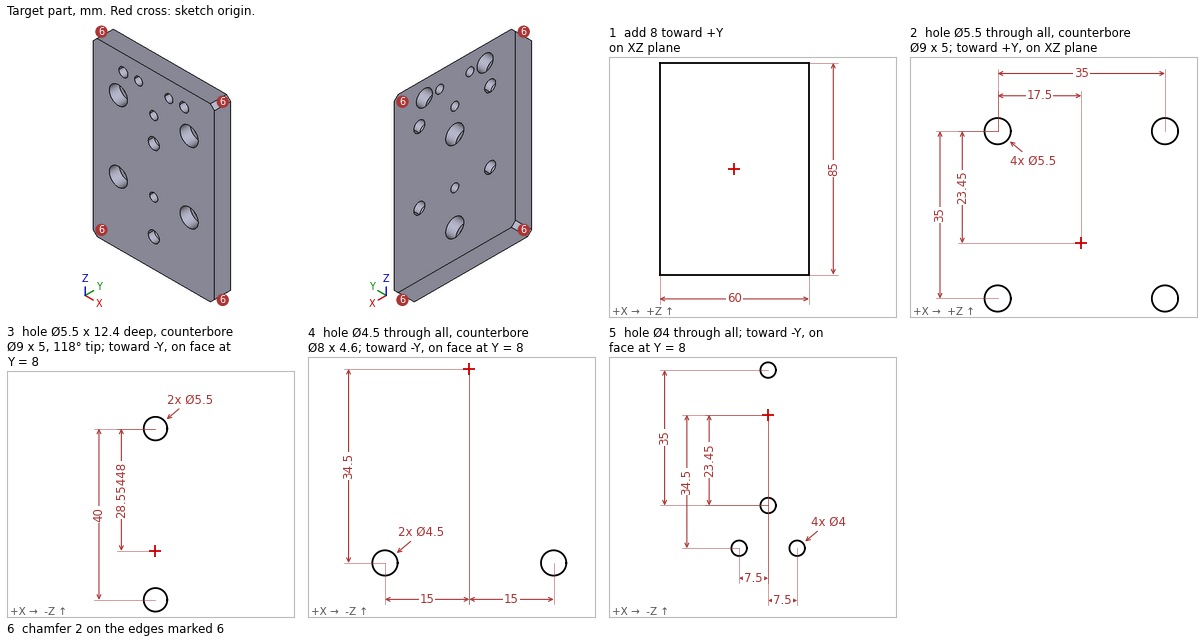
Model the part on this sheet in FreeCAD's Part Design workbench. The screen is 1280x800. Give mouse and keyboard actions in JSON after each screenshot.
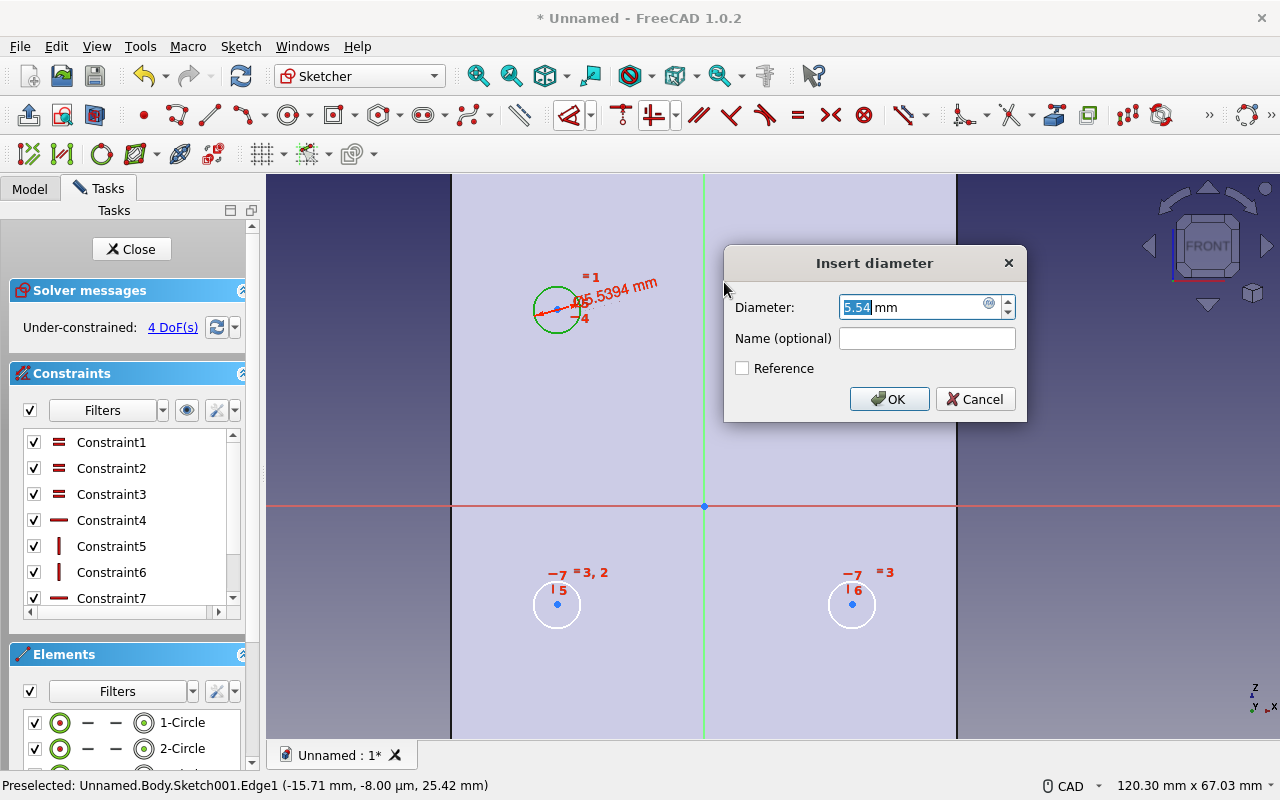
{"action": "type", "text": "5.5"}
{"action": "key", "text": "Return"}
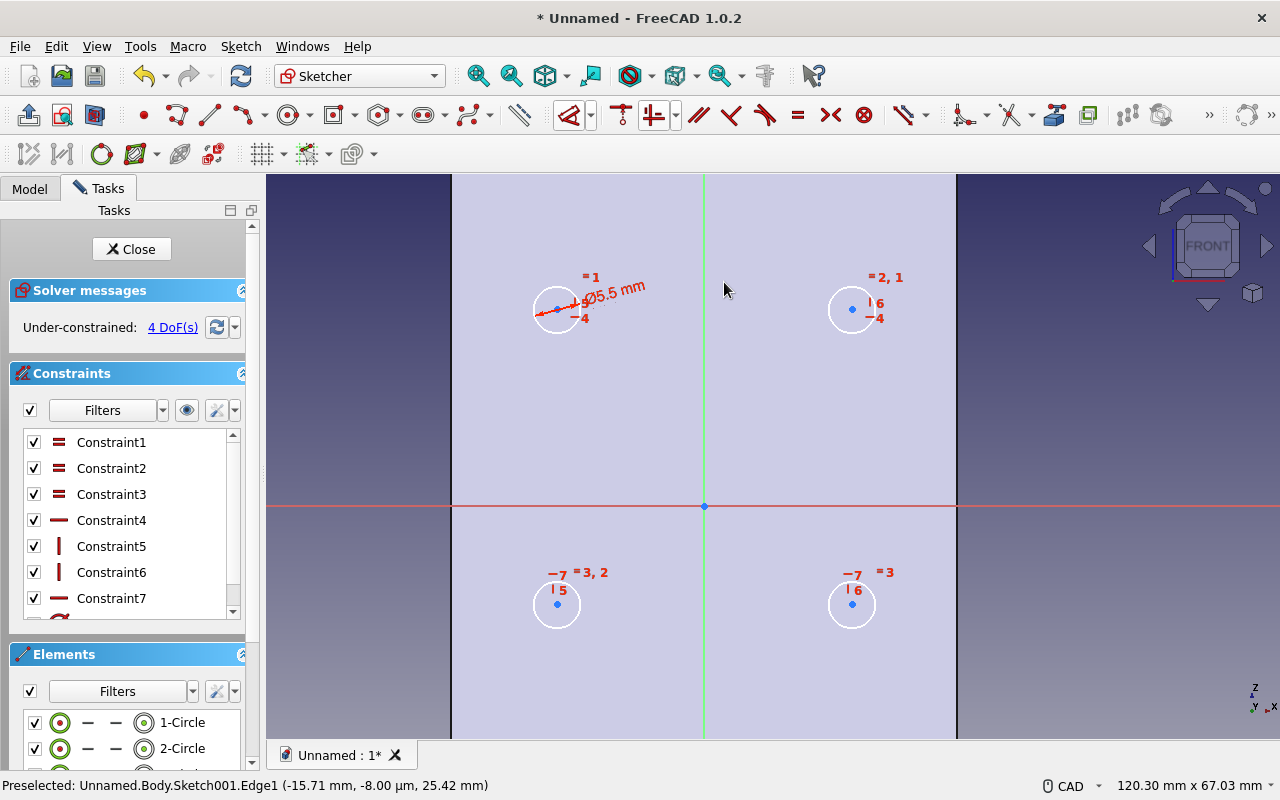
{"action": "left_click", "coordinate": [557, 310]}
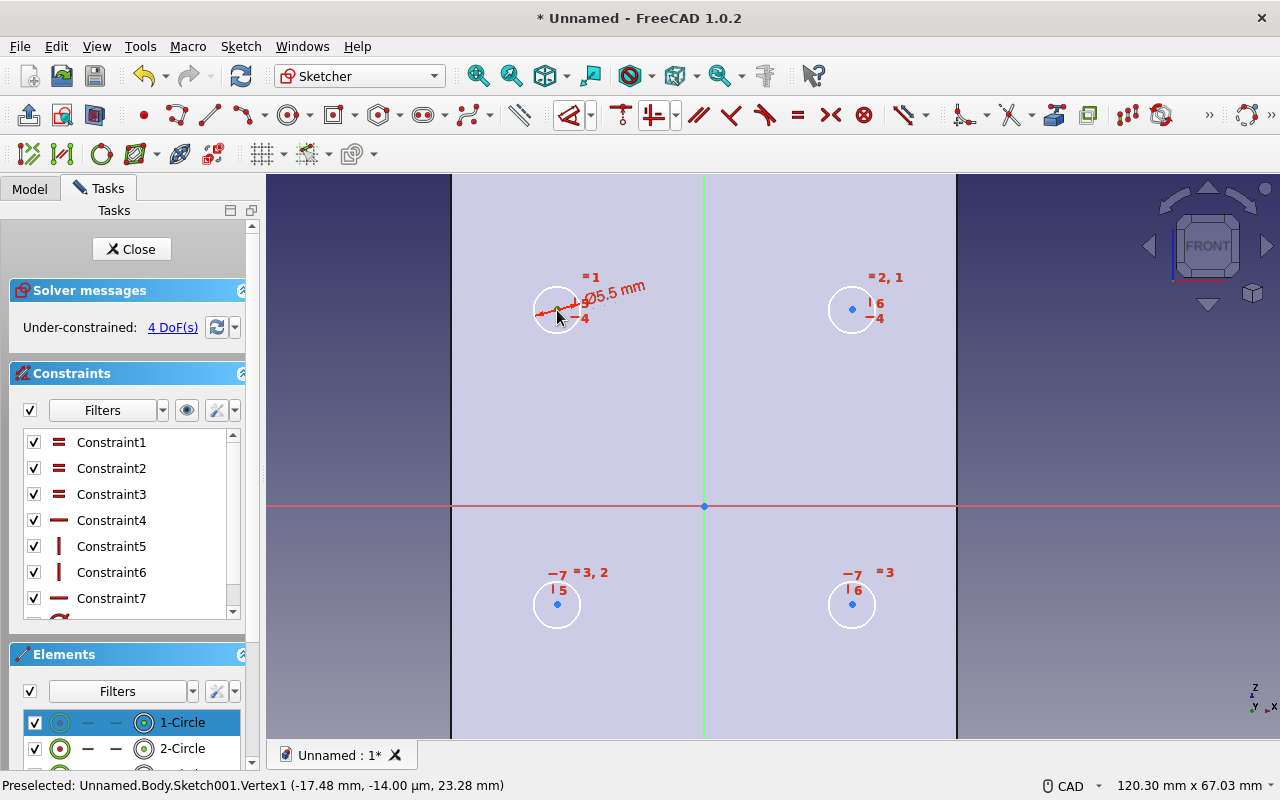
{"action": "left_click", "coordinate": [852, 310]}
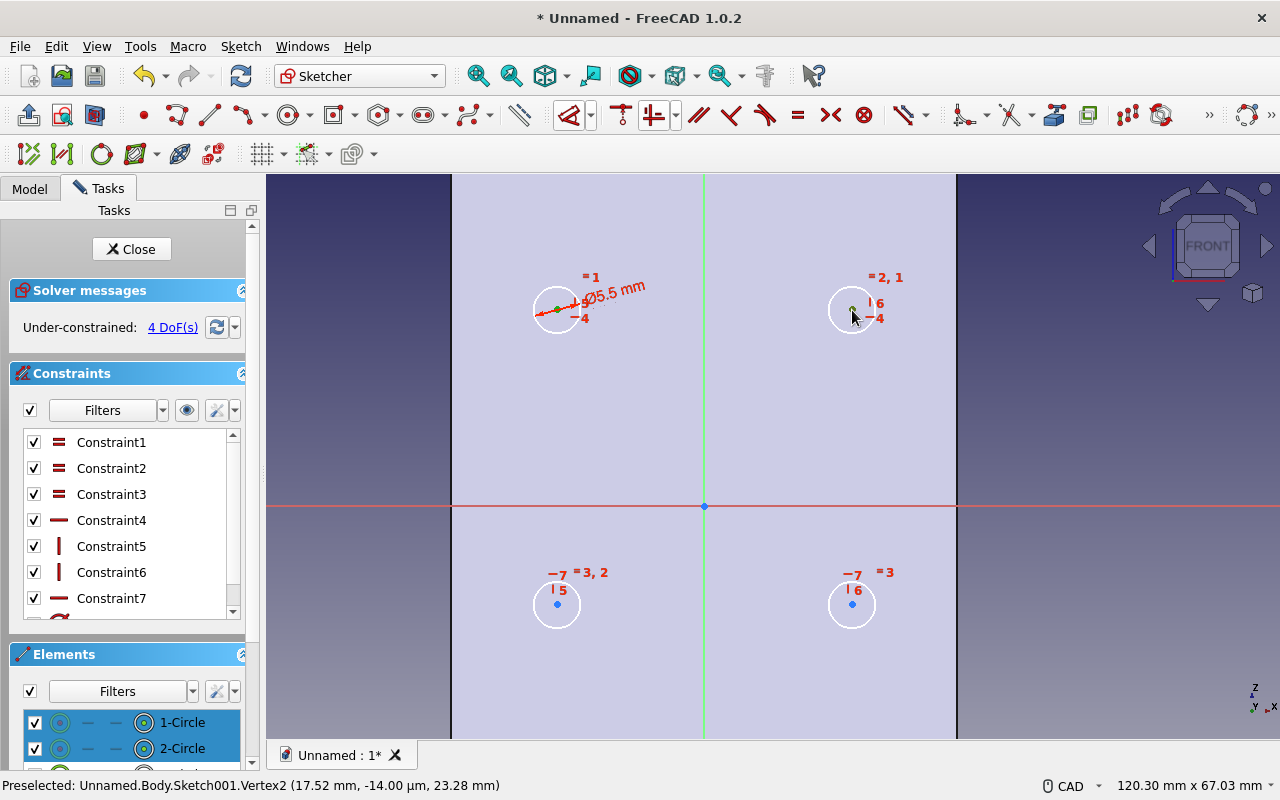
{"action": "key", "text": "l"}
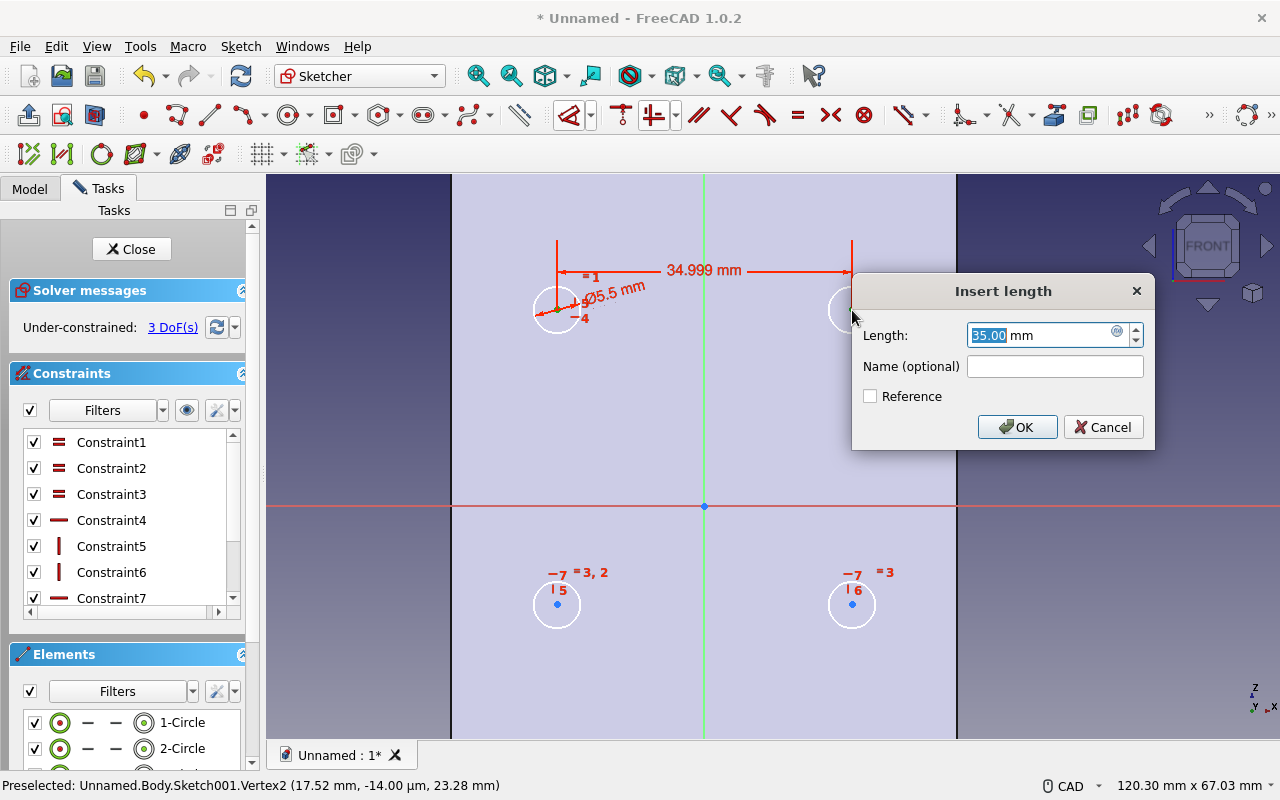
{"action": "type", "text": "35"}
{"action": "key", "text": "Return"}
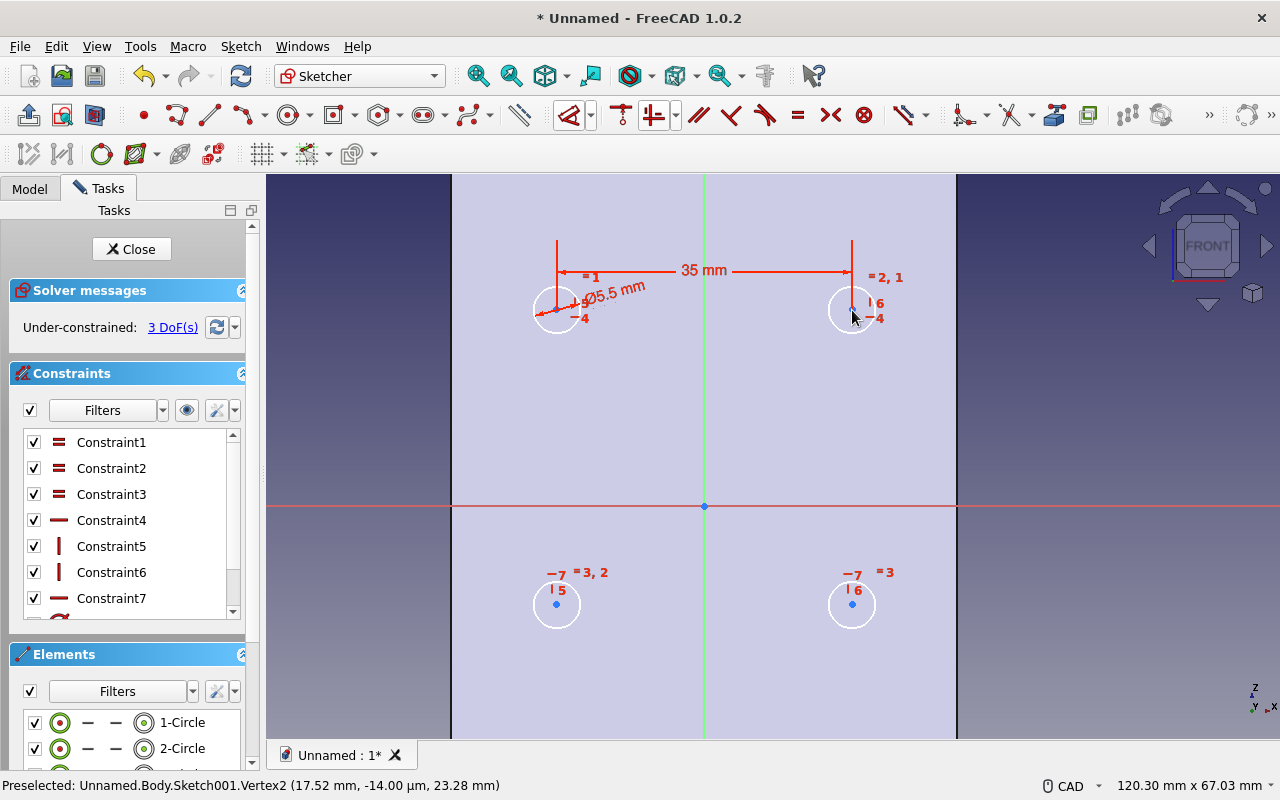
{"action": "left_click", "coordinate": [557, 310]}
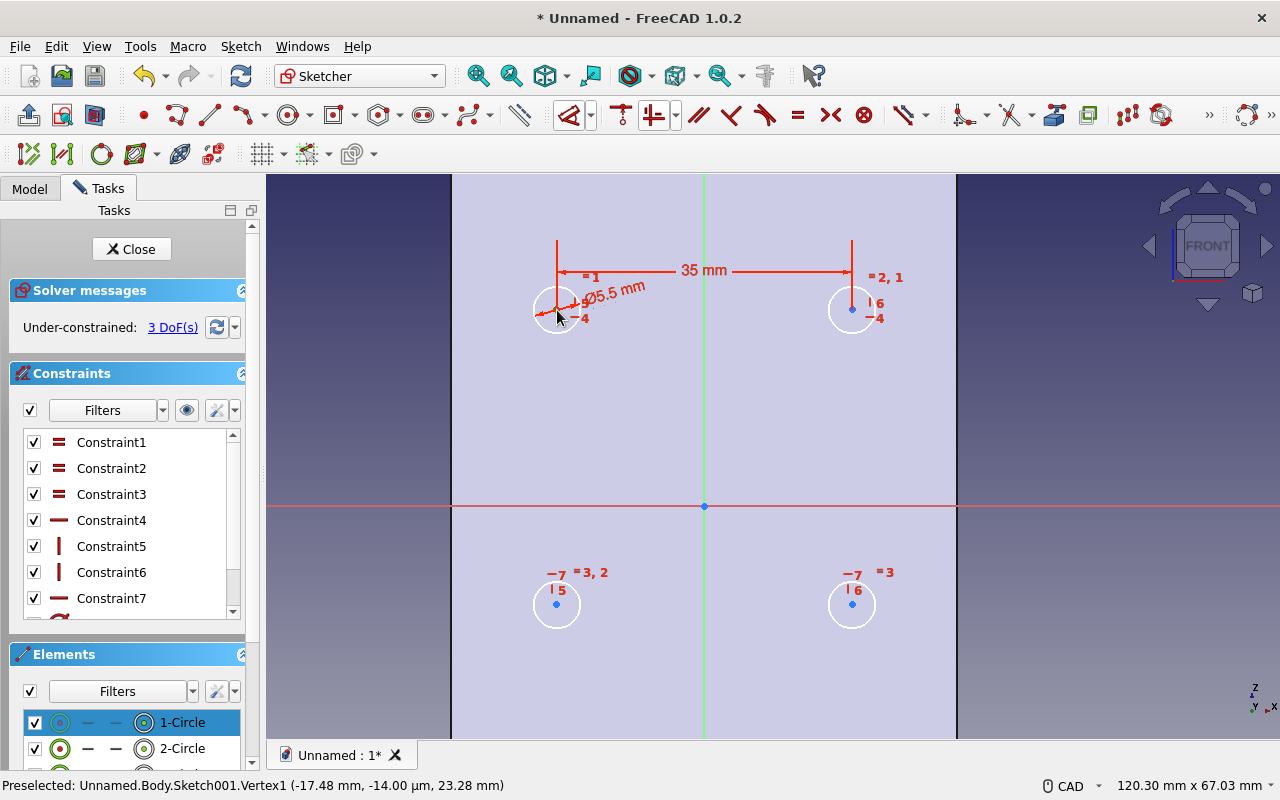
{"action": "left_click", "coordinate": [557, 605]}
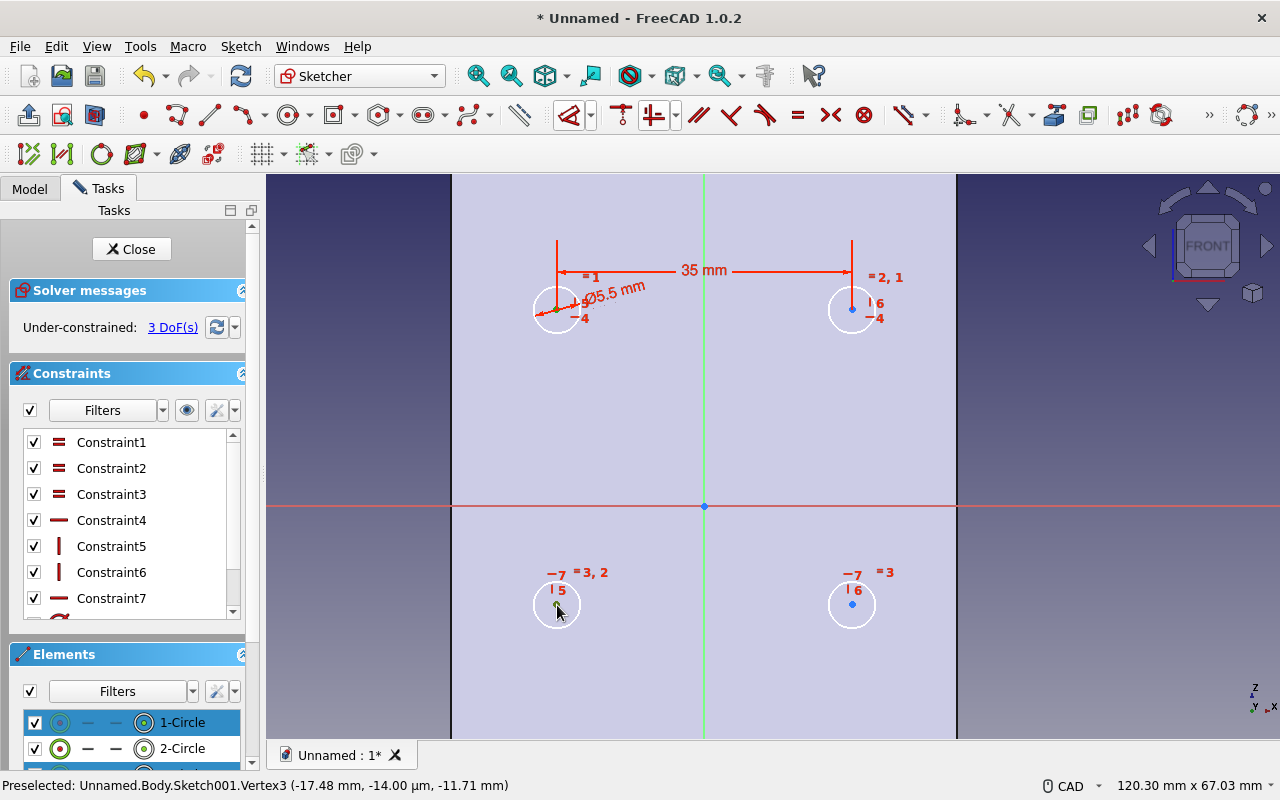
{"action": "left_click", "coordinate": [590, 116]}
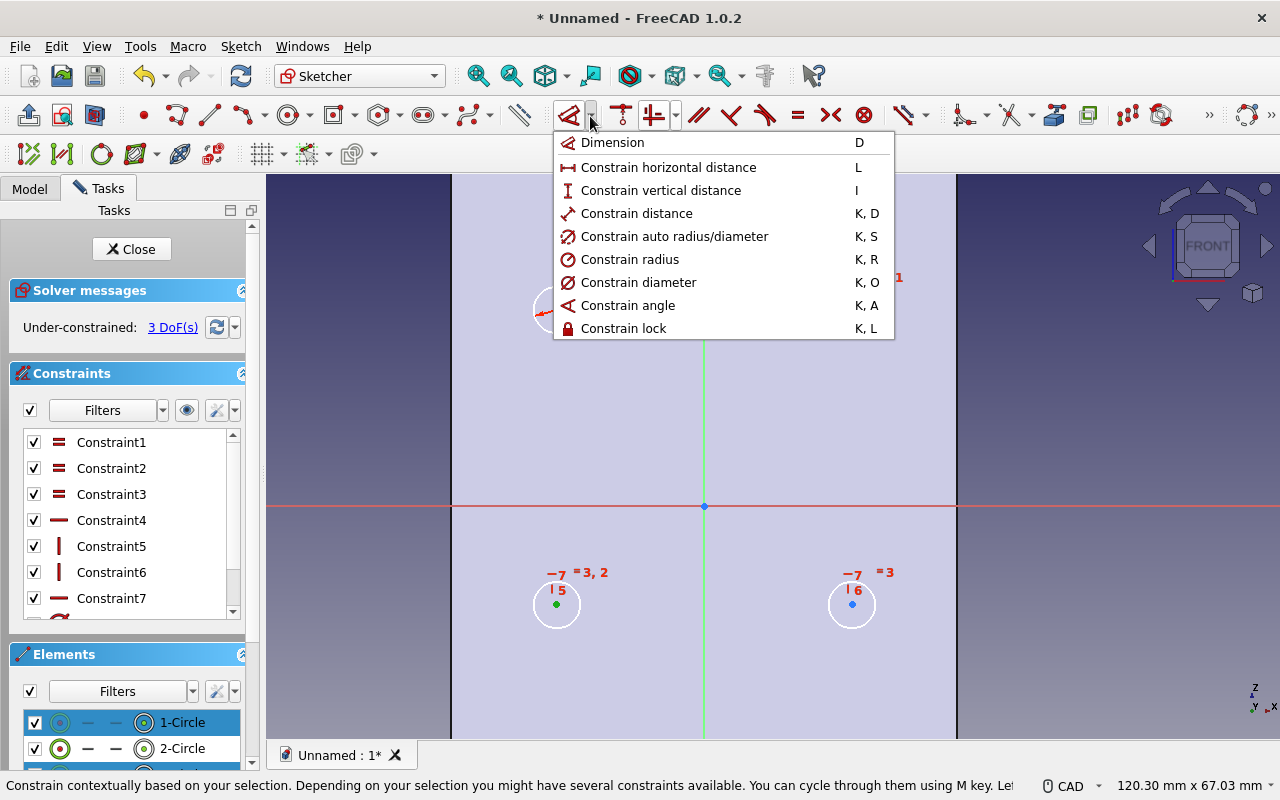
{"action": "left_click", "coordinate": [724, 190]}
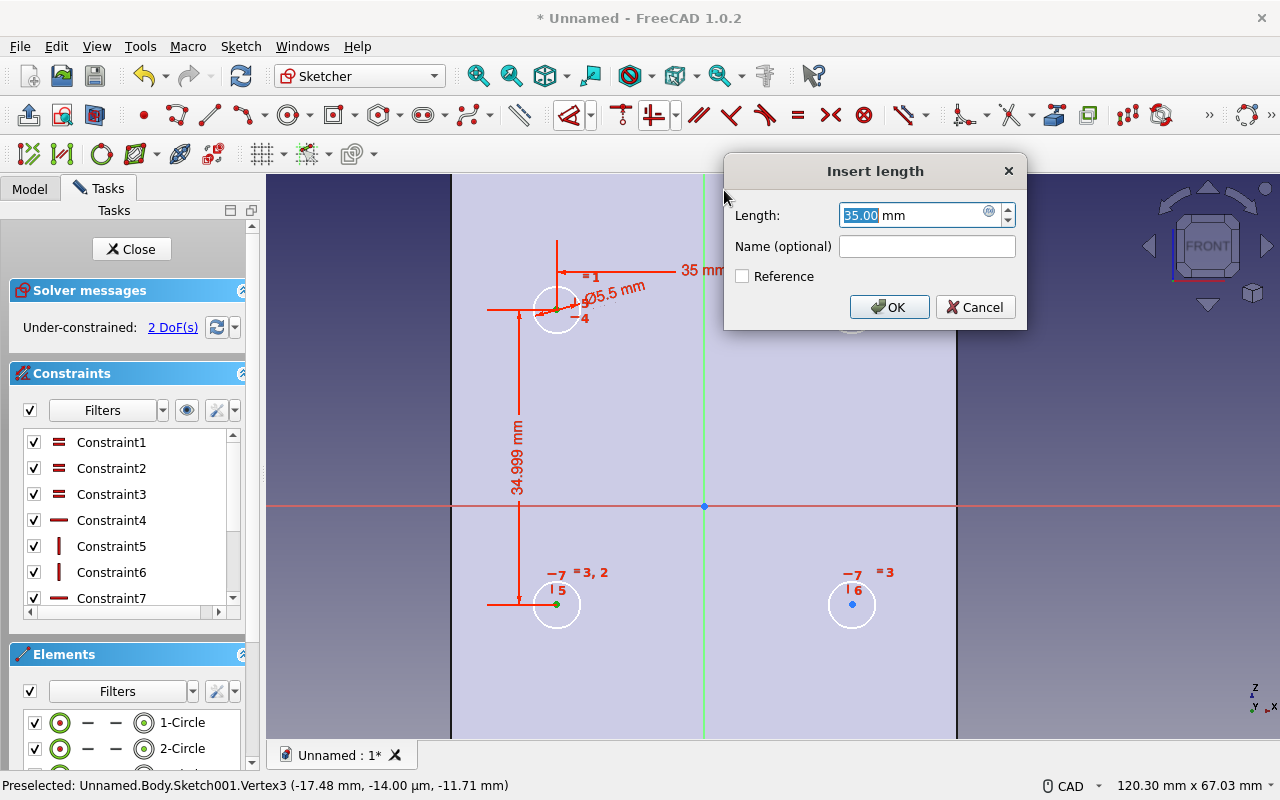
{"action": "type", "text": "35"}
{"action": "key", "text": "Return"}